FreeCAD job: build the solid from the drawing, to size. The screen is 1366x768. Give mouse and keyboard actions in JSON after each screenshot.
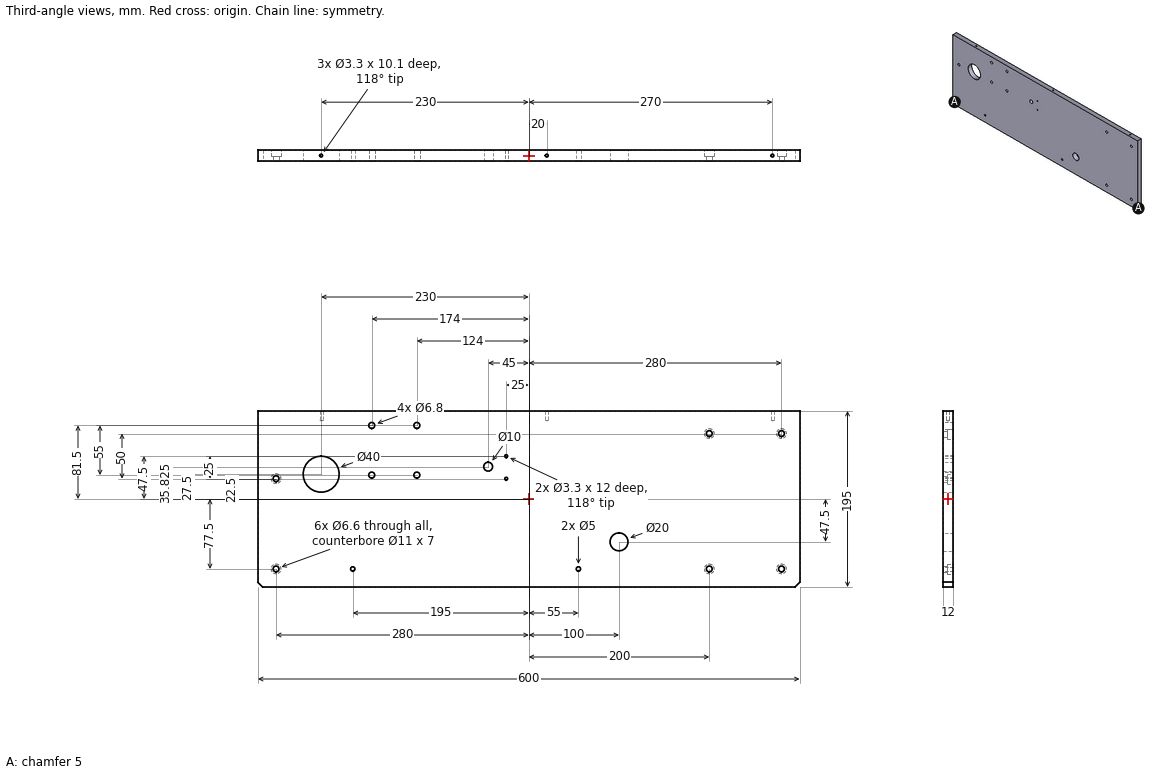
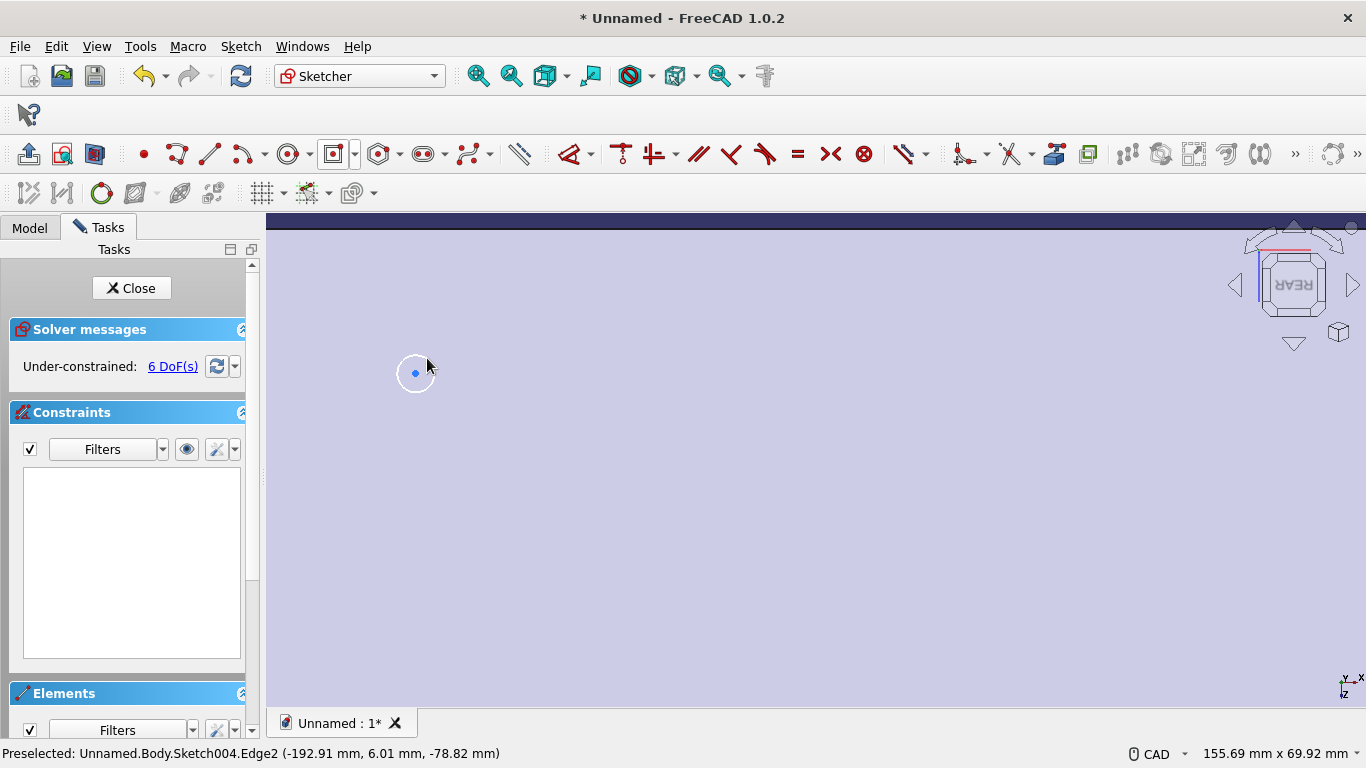
{"action": "scroll", "coordinate": [427, 358], "scroll_direction": "down", "scroll_amount": 5}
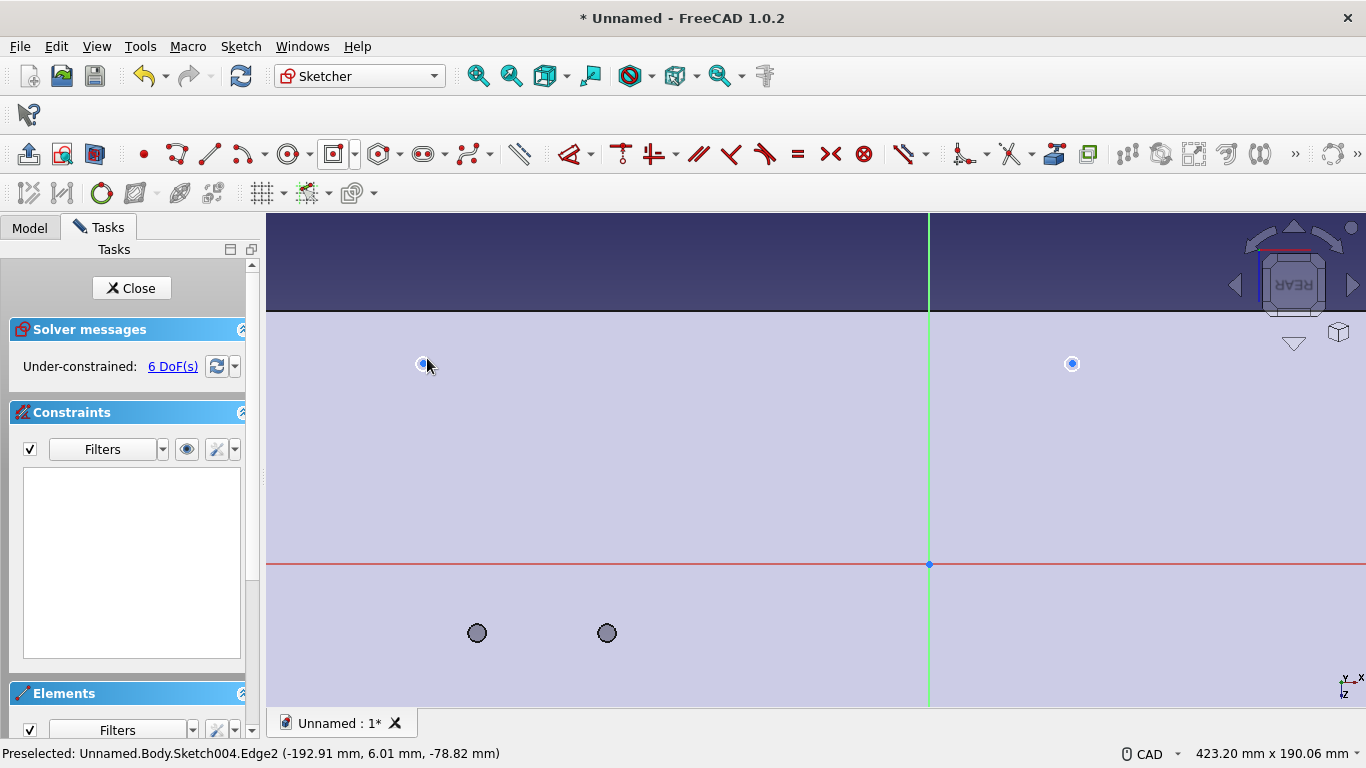
{"action": "scroll", "coordinate": [1077, 359], "scroll_direction": "up", "scroll_amount": 4}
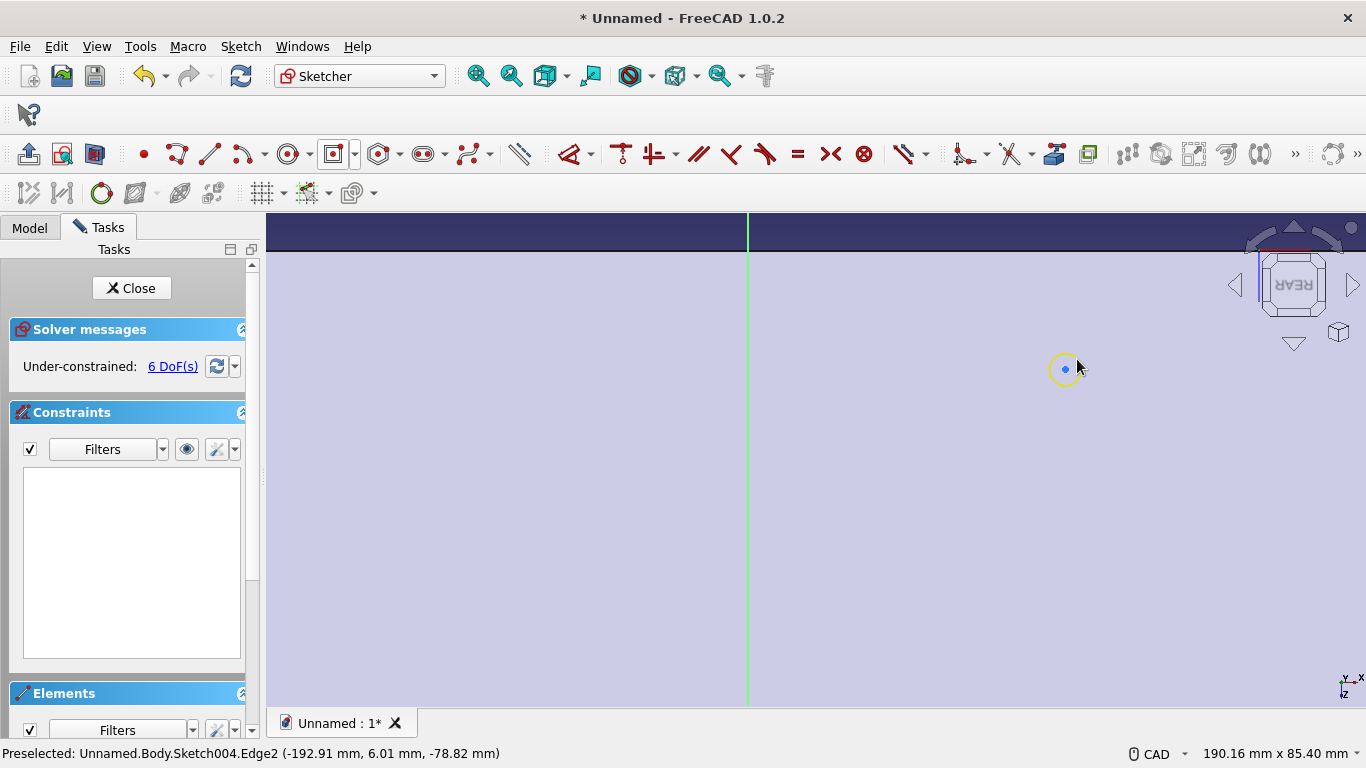
{"action": "left_click", "coordinate": [1077, 358]}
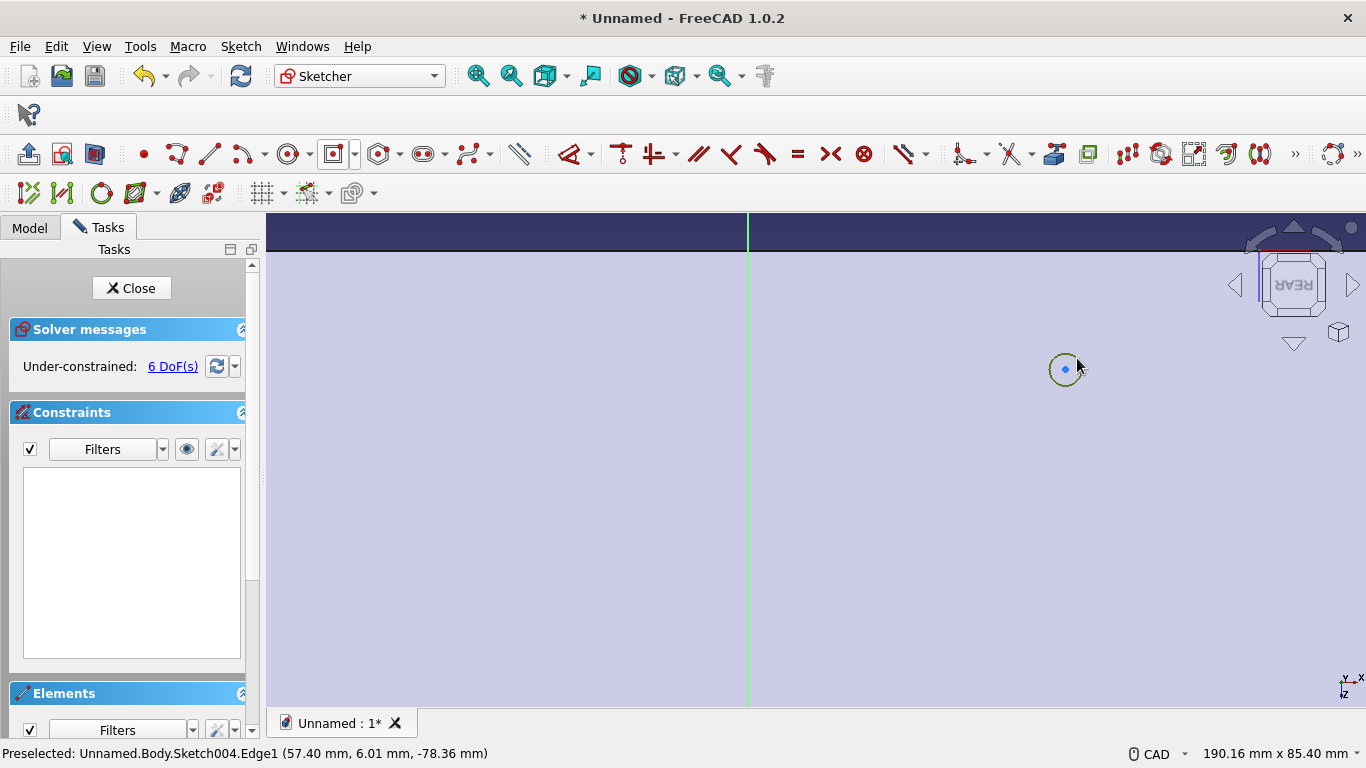
{"action": "scroll", "coordinate": [1078, 359], "scroll_direction": "down", "scroll_amount": 4}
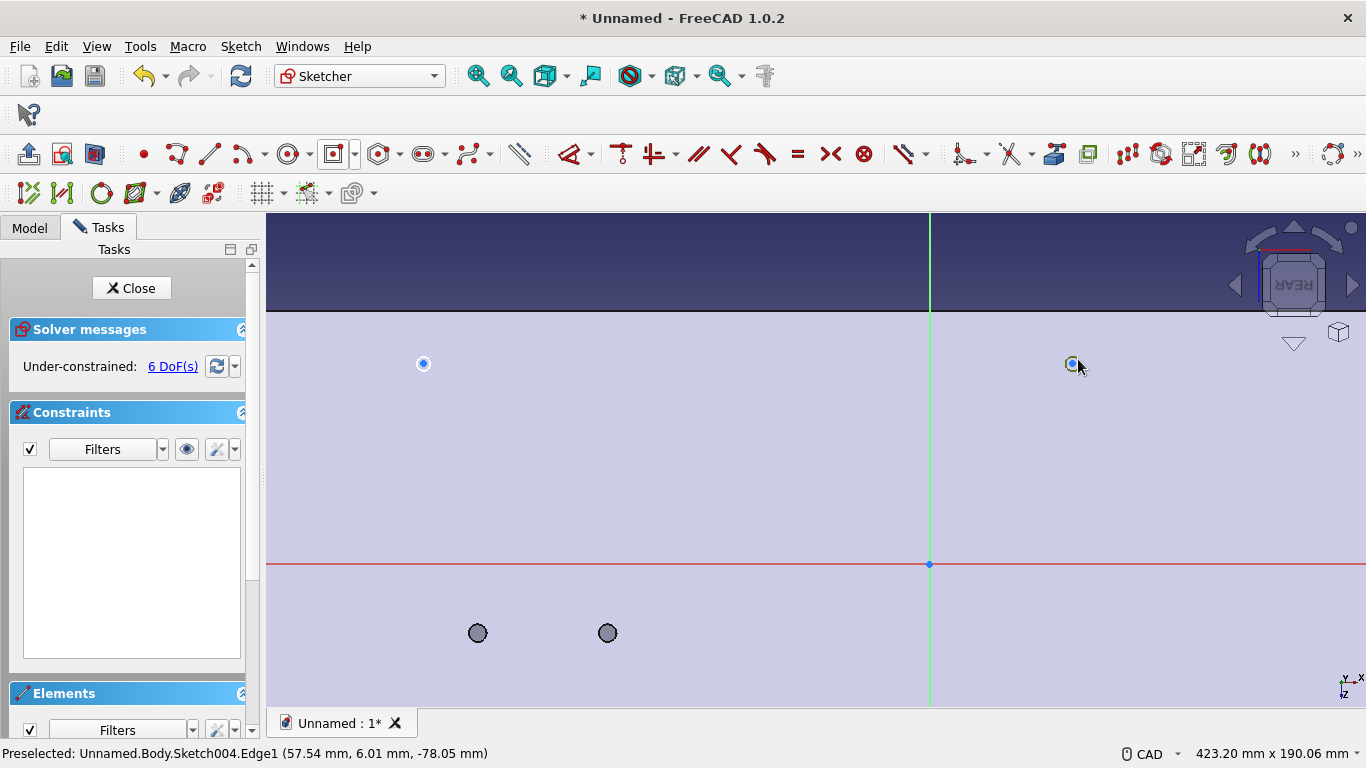
{"action": "scroll", "coordinate": [428, 359], "scroll_direction": "up", "scroll_amount": 4}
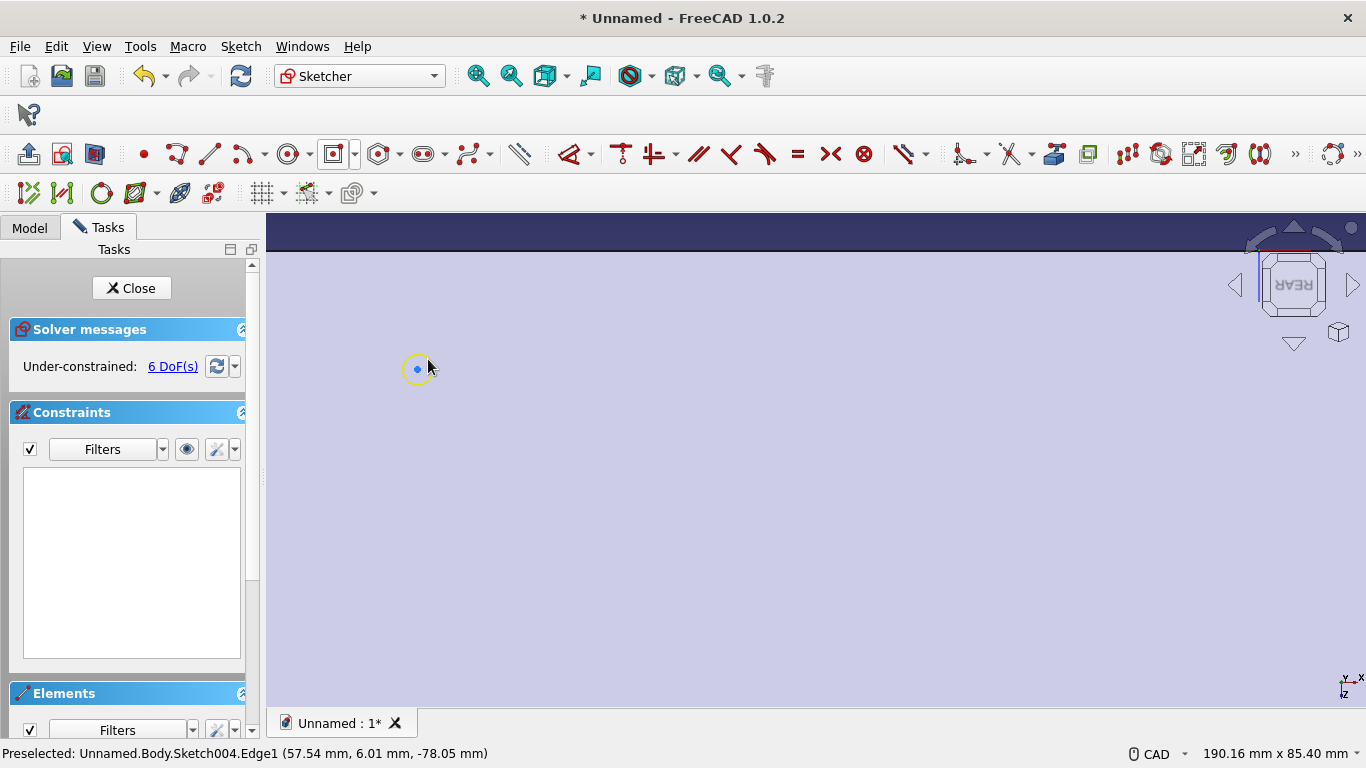
{"action": "left_click", "coordinate": [429, 359]}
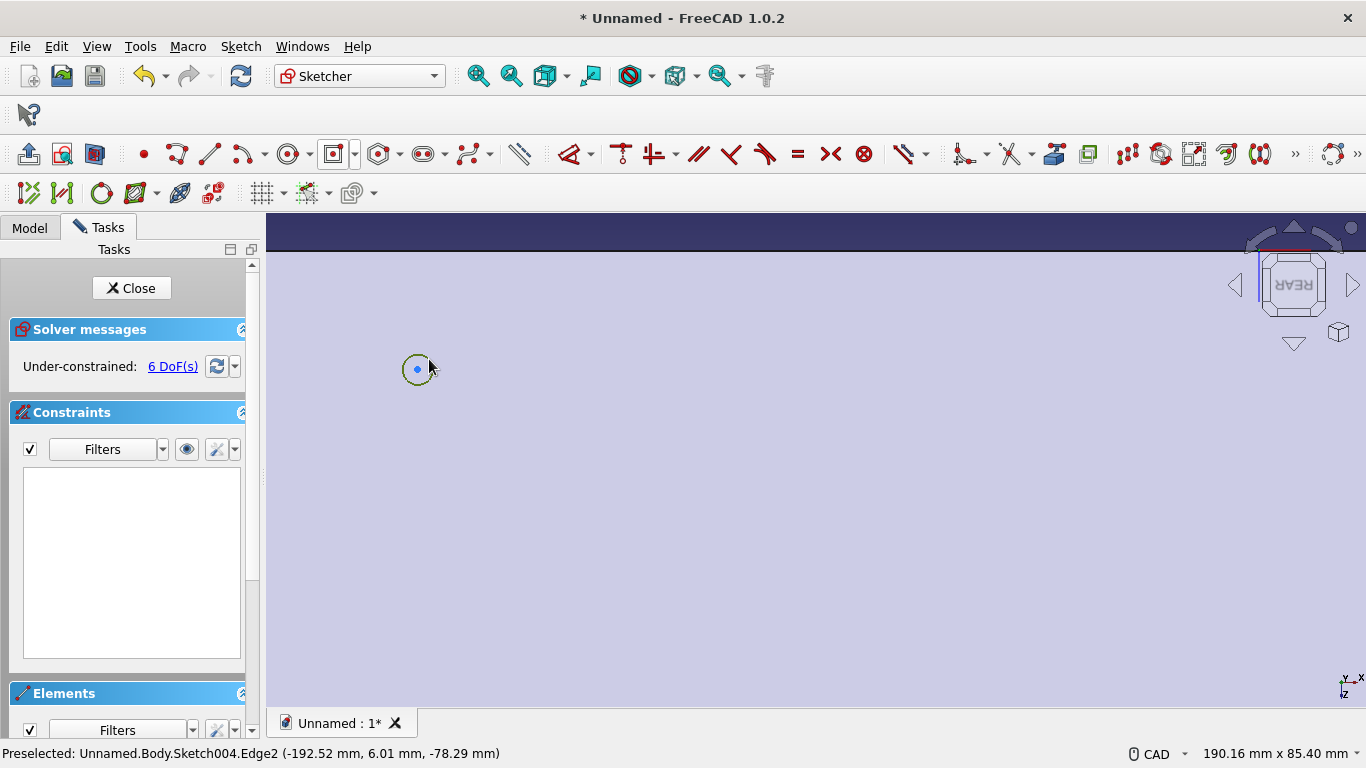
{"action": "key", "text": "e"}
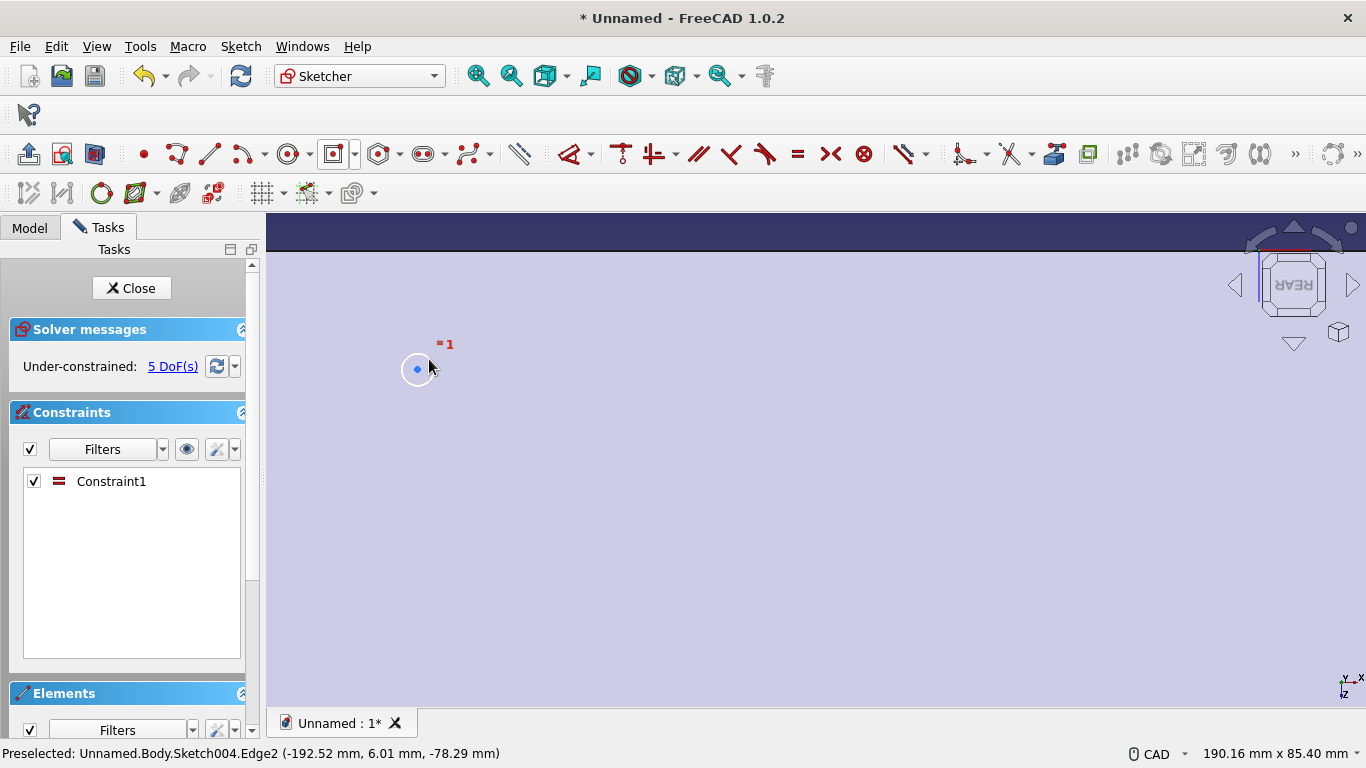
{"action": "key", "text": "d"}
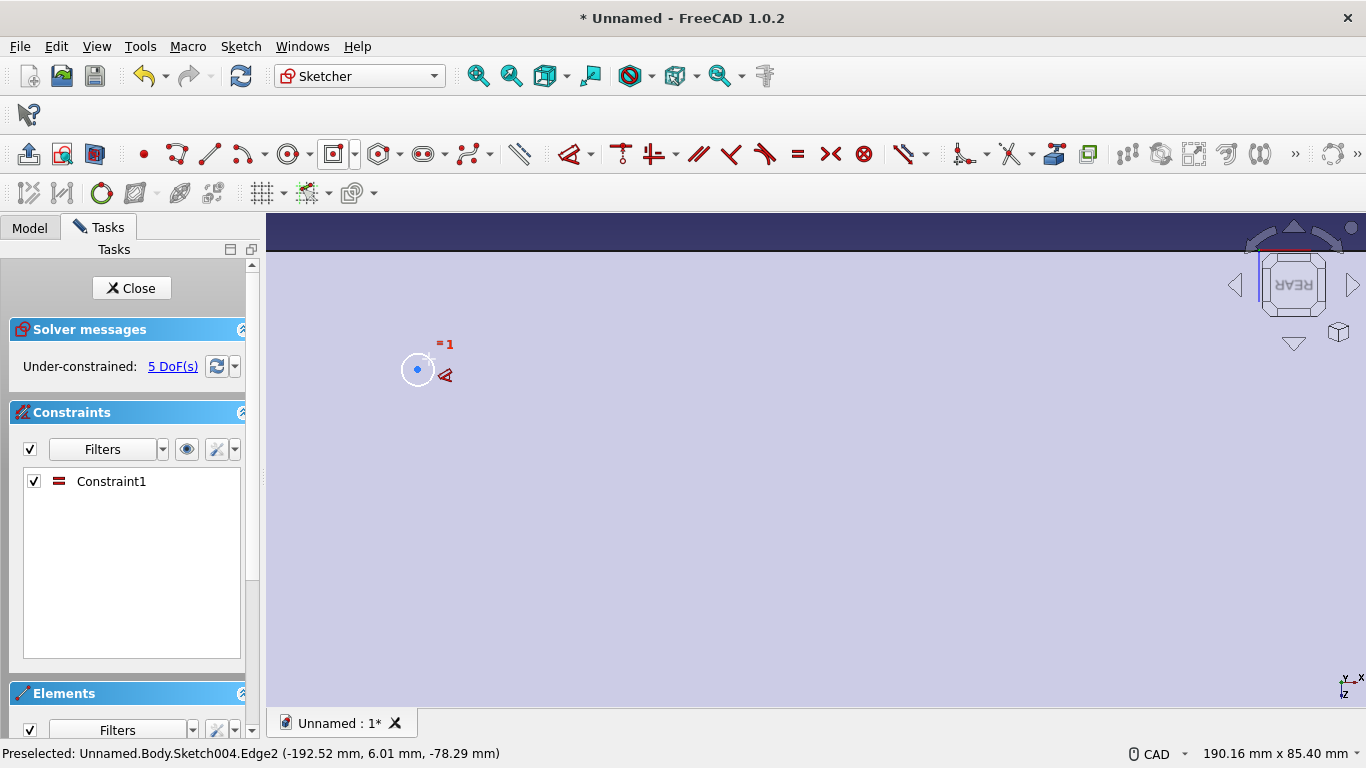
{"action": "scroll", "coordinate": [427, 359], "scroll_direction": "down", "scroll_amount": 4}